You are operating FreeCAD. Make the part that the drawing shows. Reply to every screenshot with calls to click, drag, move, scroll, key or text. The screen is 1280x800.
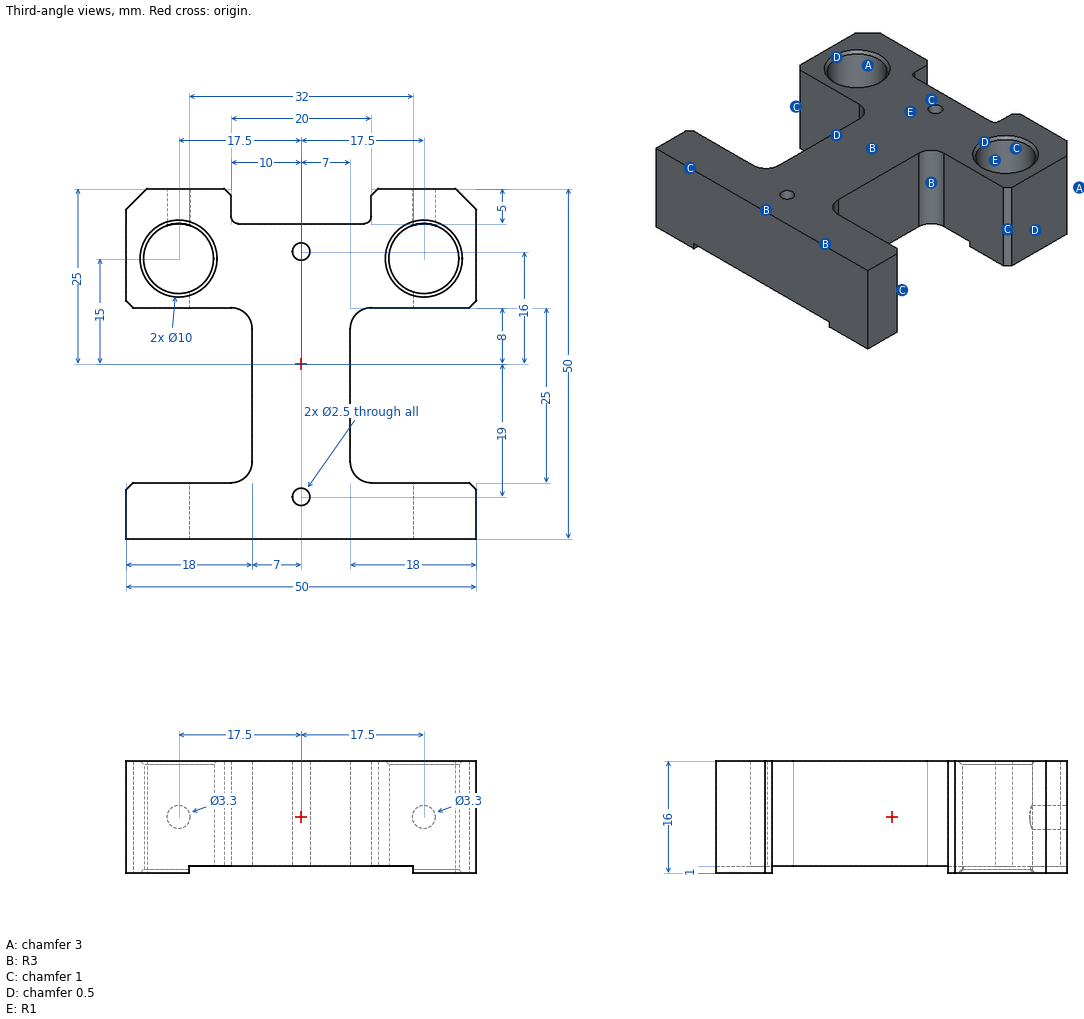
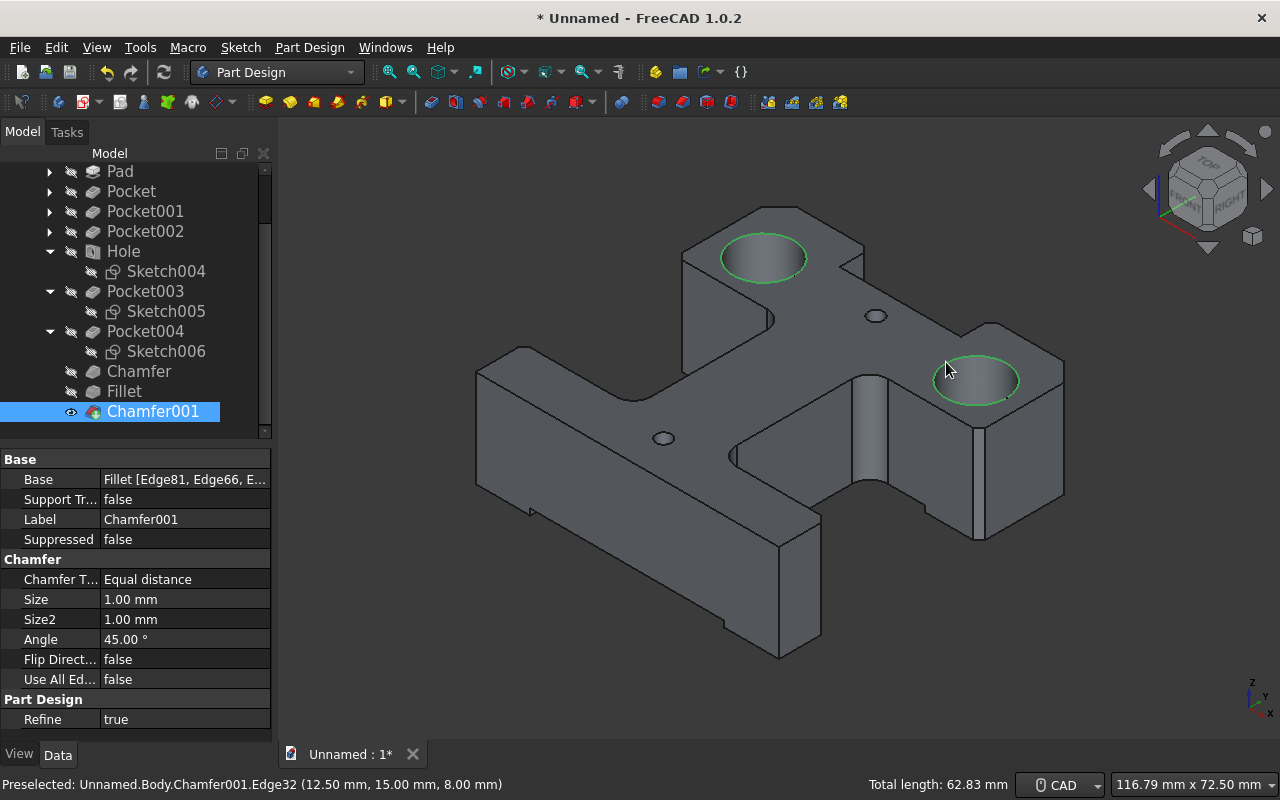
key(2)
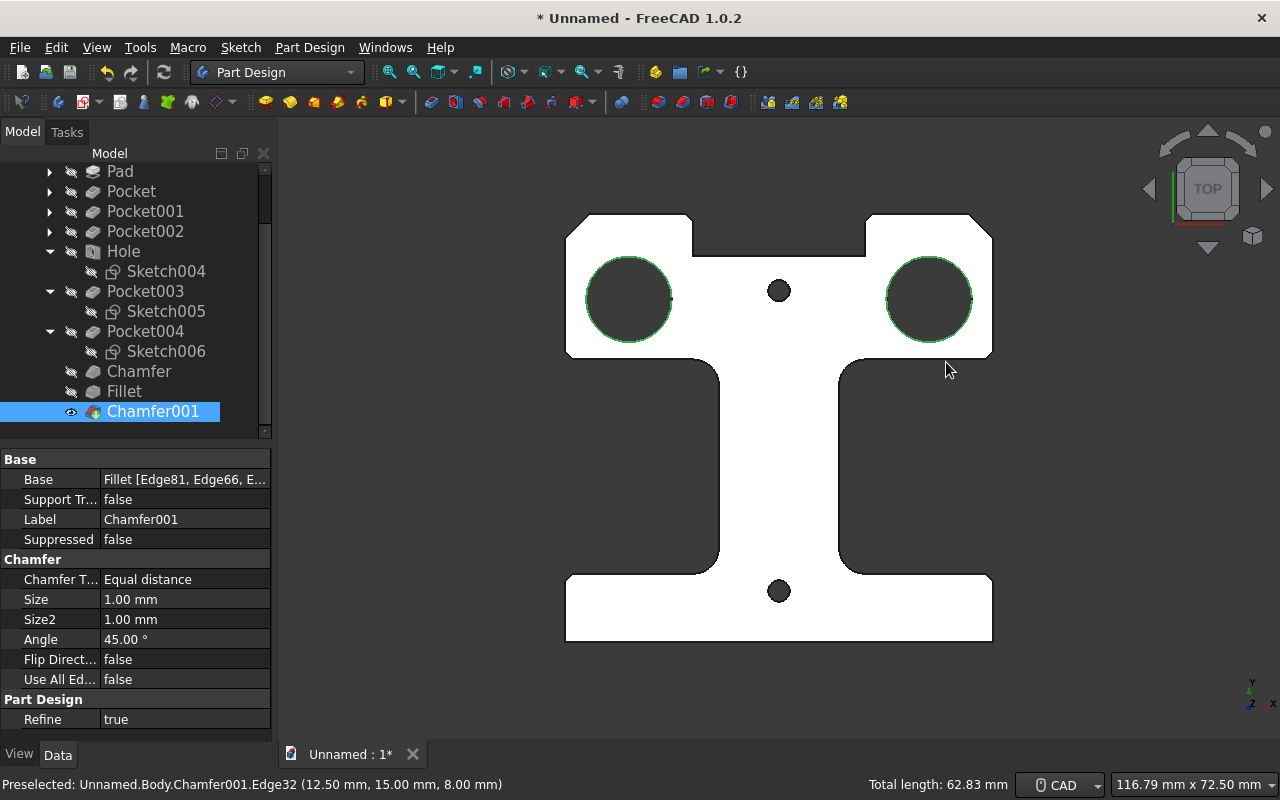
key(1)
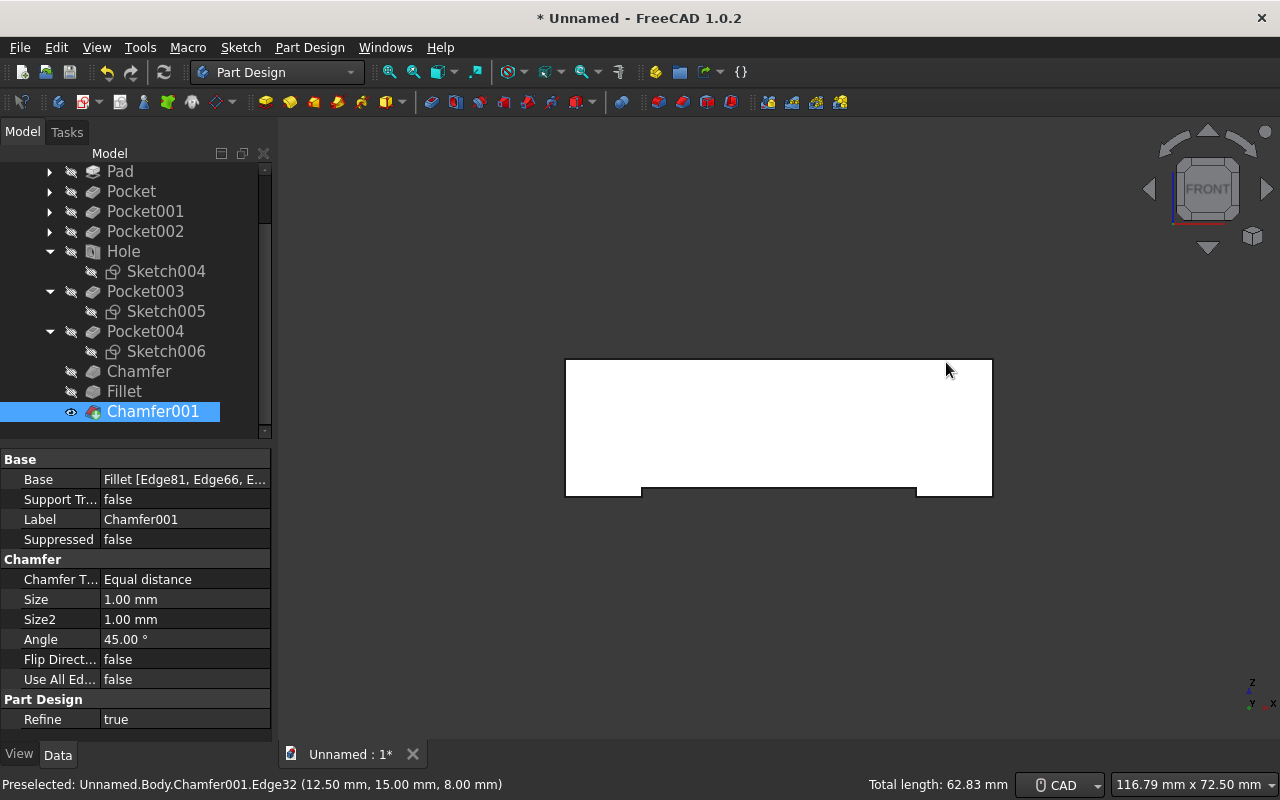
key(v)
key(f)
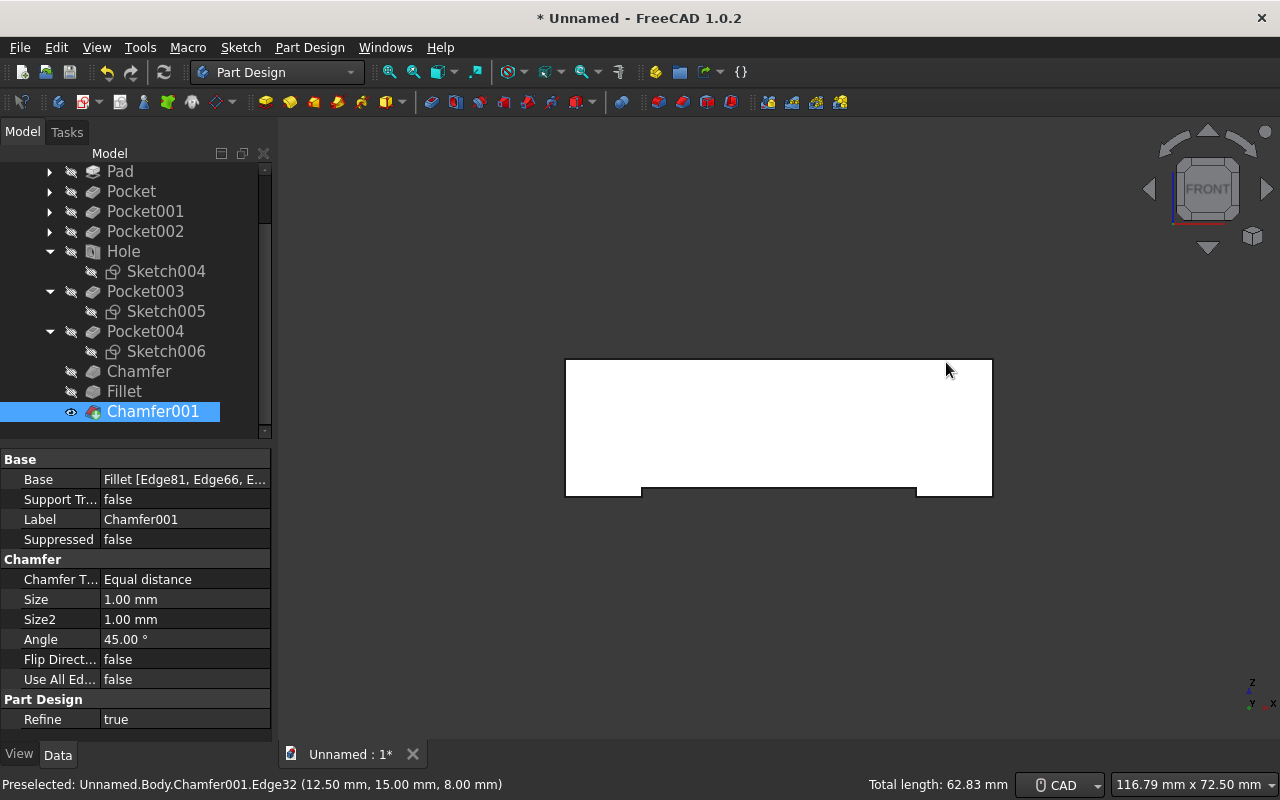
key(3)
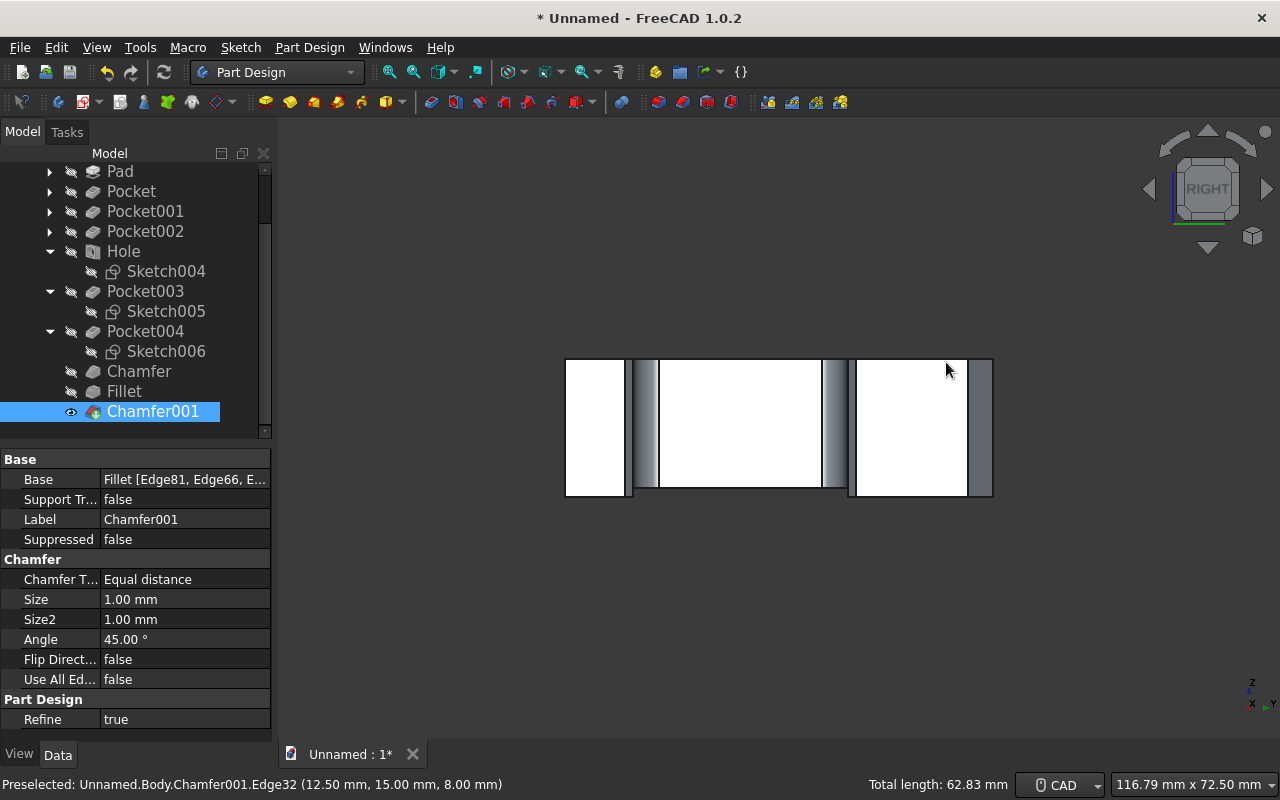
click(390, 72)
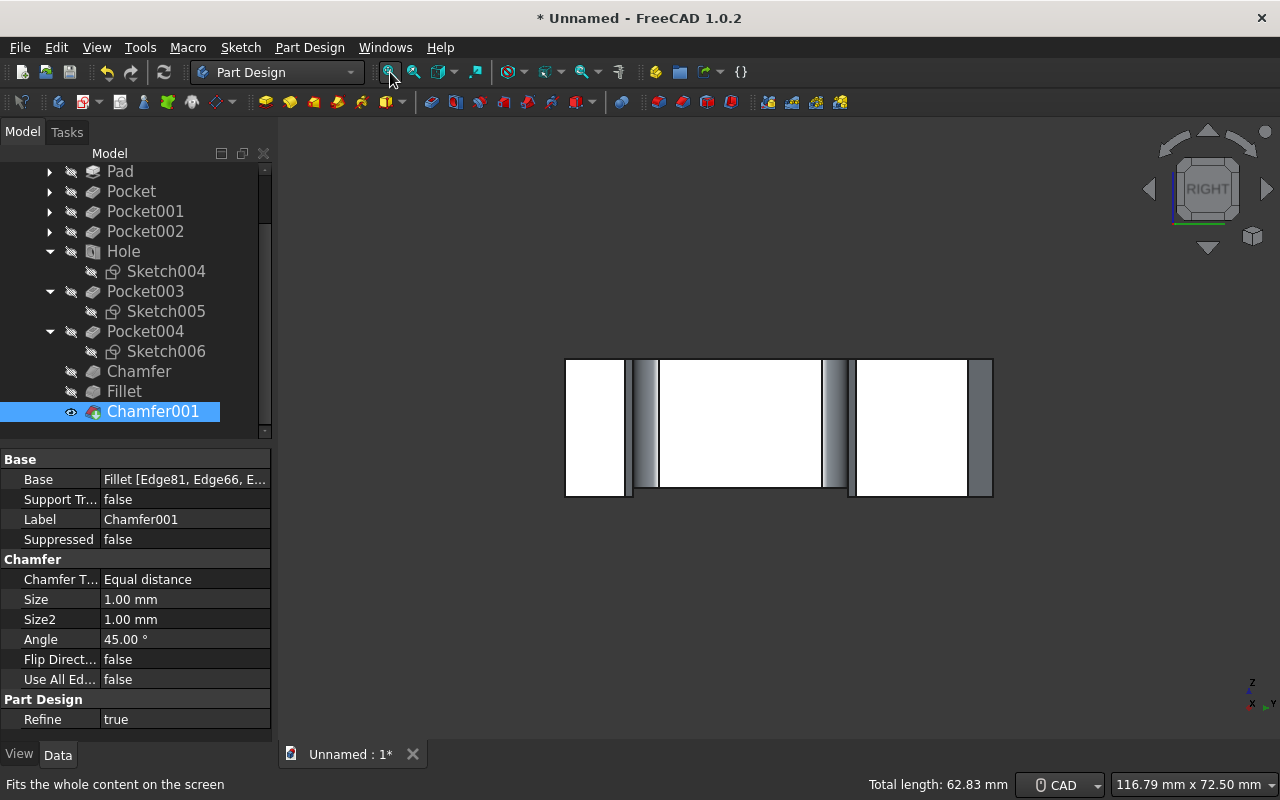
key(5)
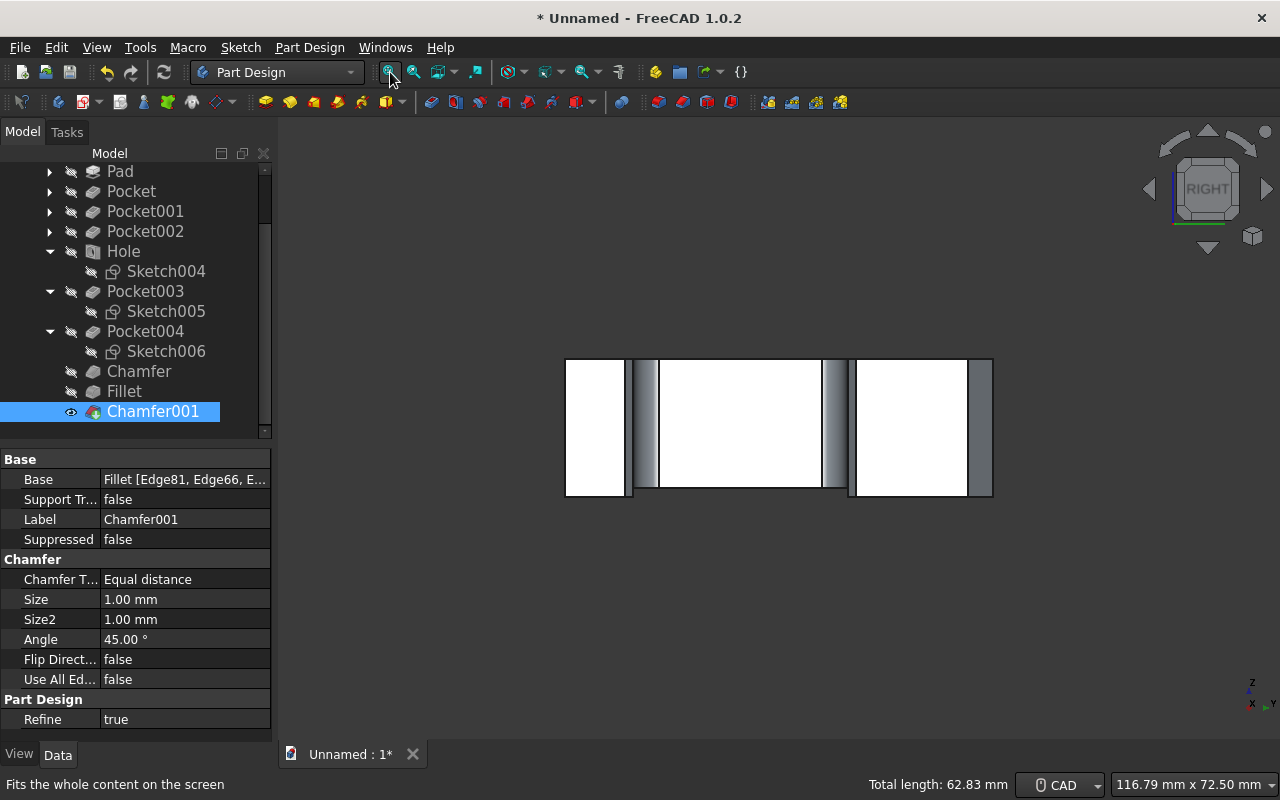
click(586, 556, ctrl)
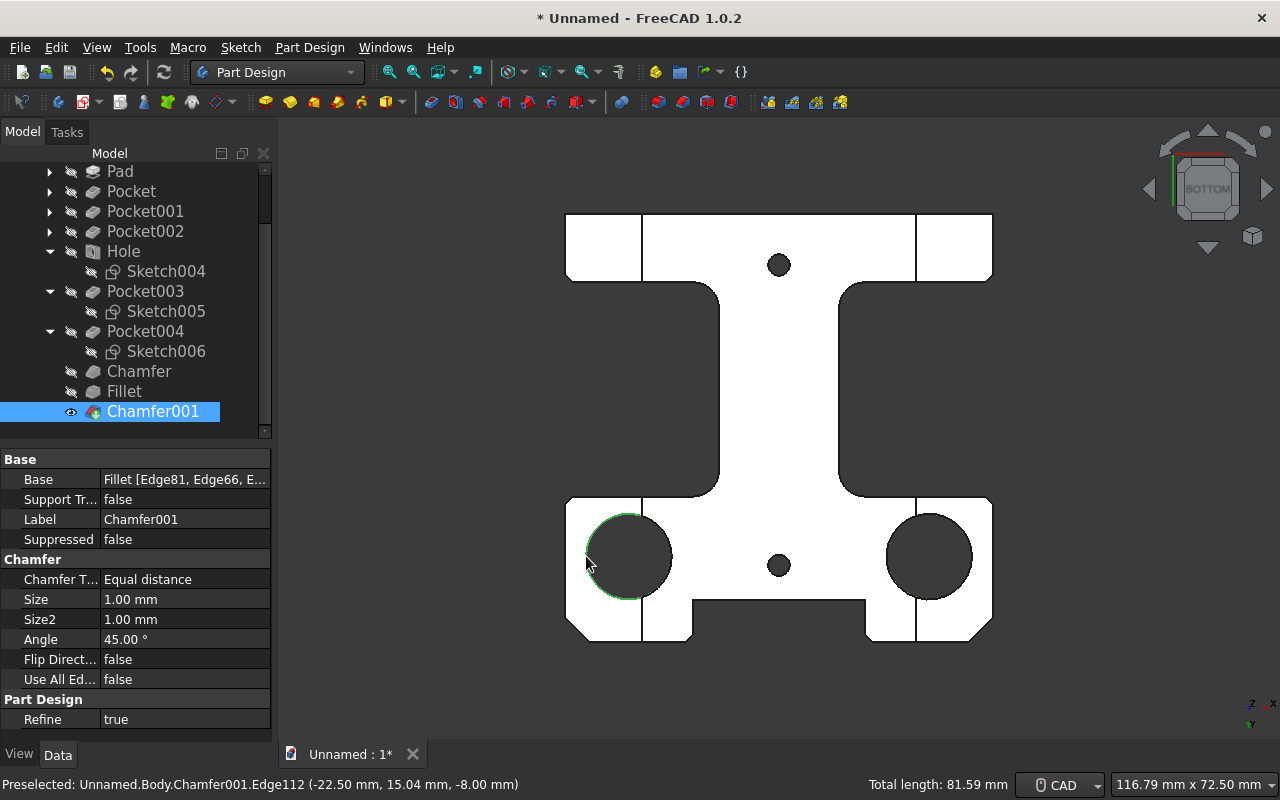
click(955, 590, ctrl)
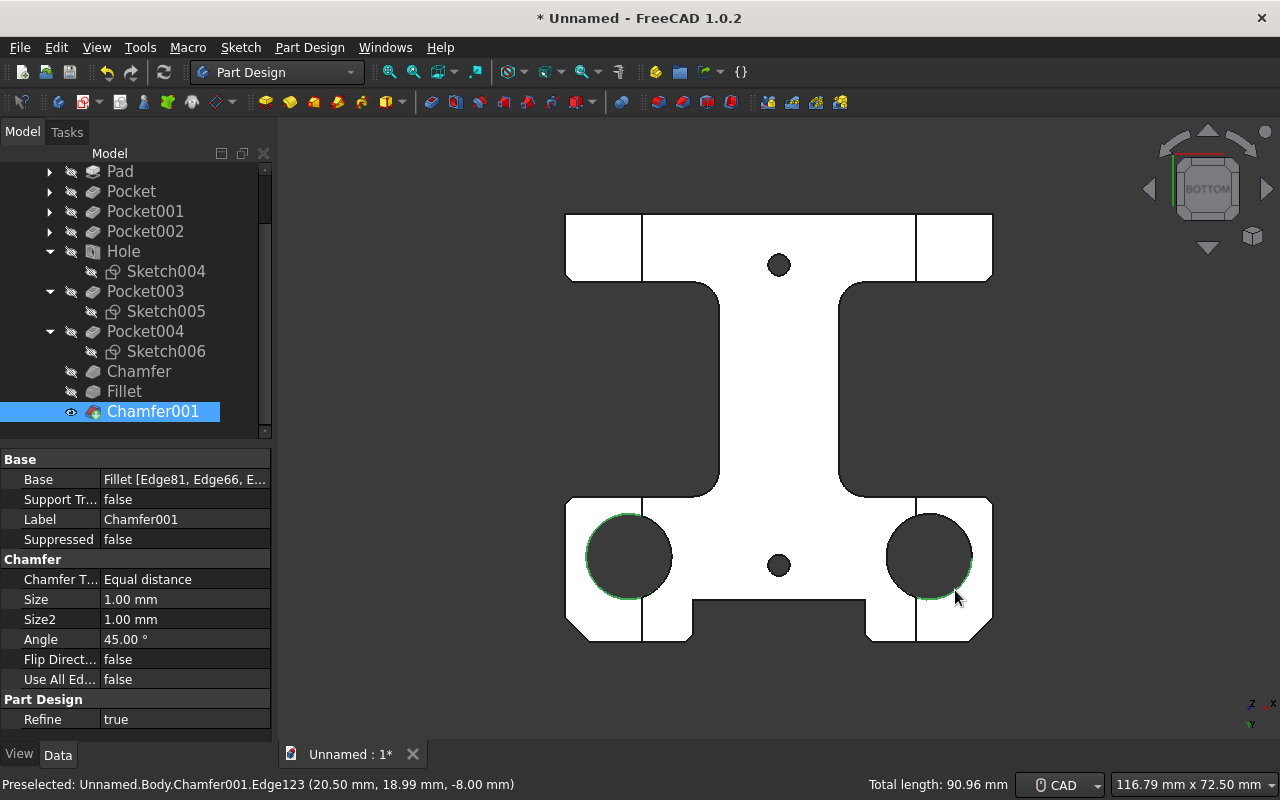
click(684, 102)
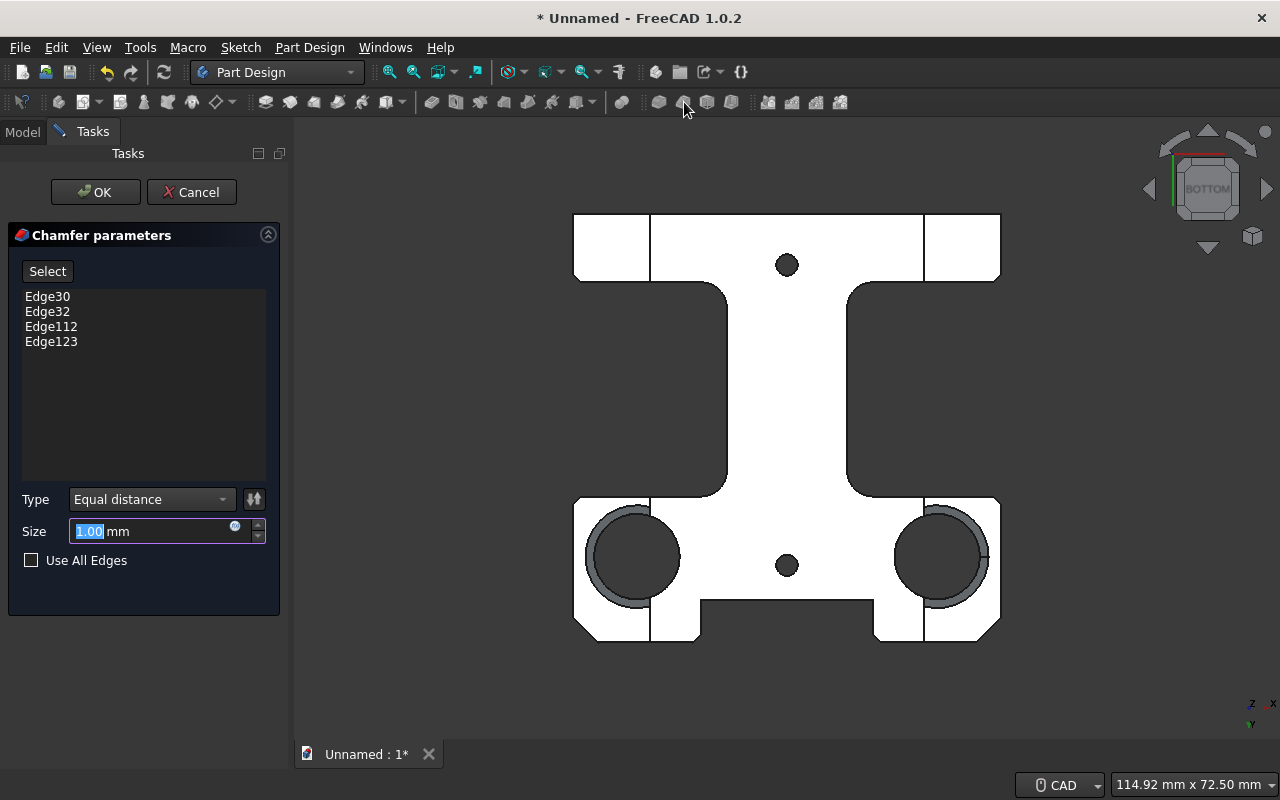
text(0.5)
key(Tab)